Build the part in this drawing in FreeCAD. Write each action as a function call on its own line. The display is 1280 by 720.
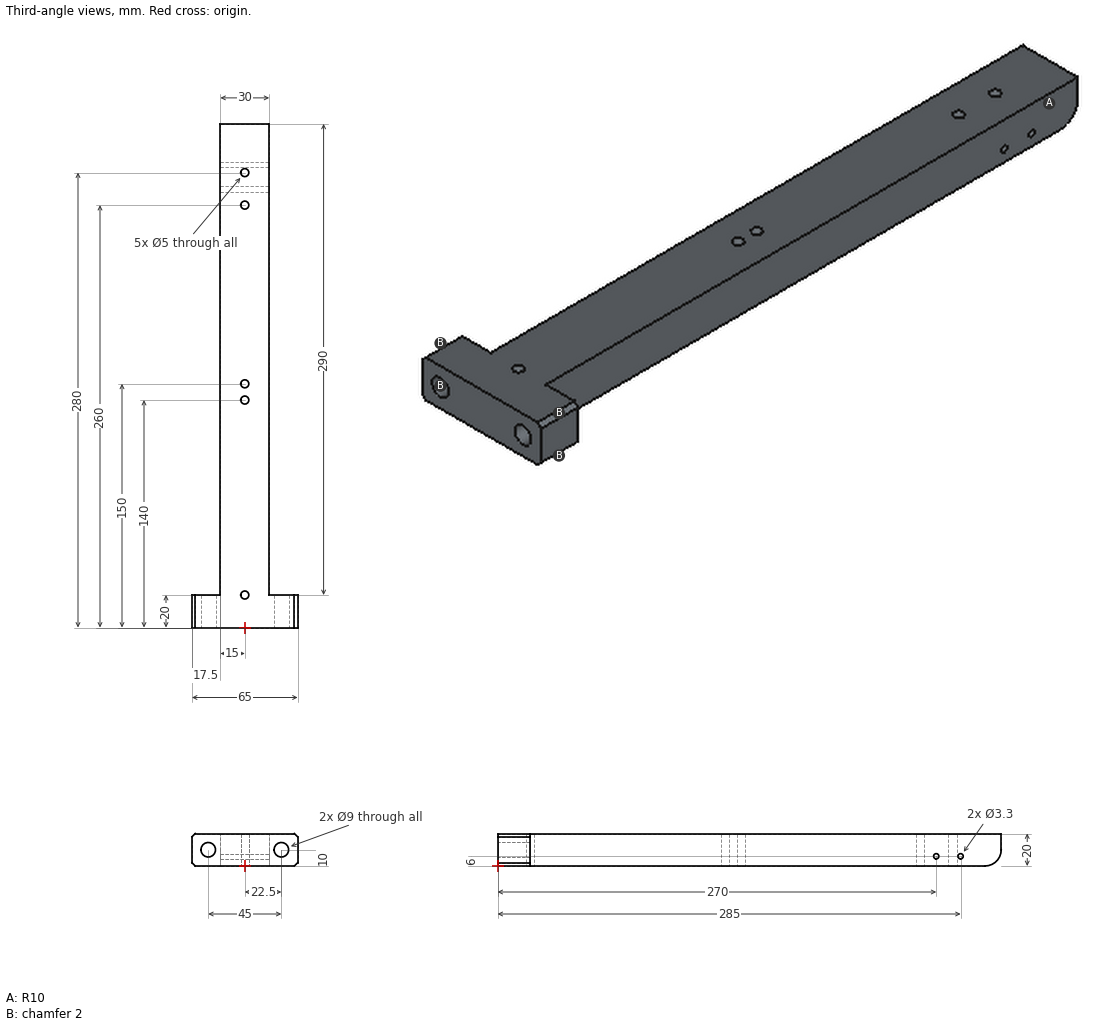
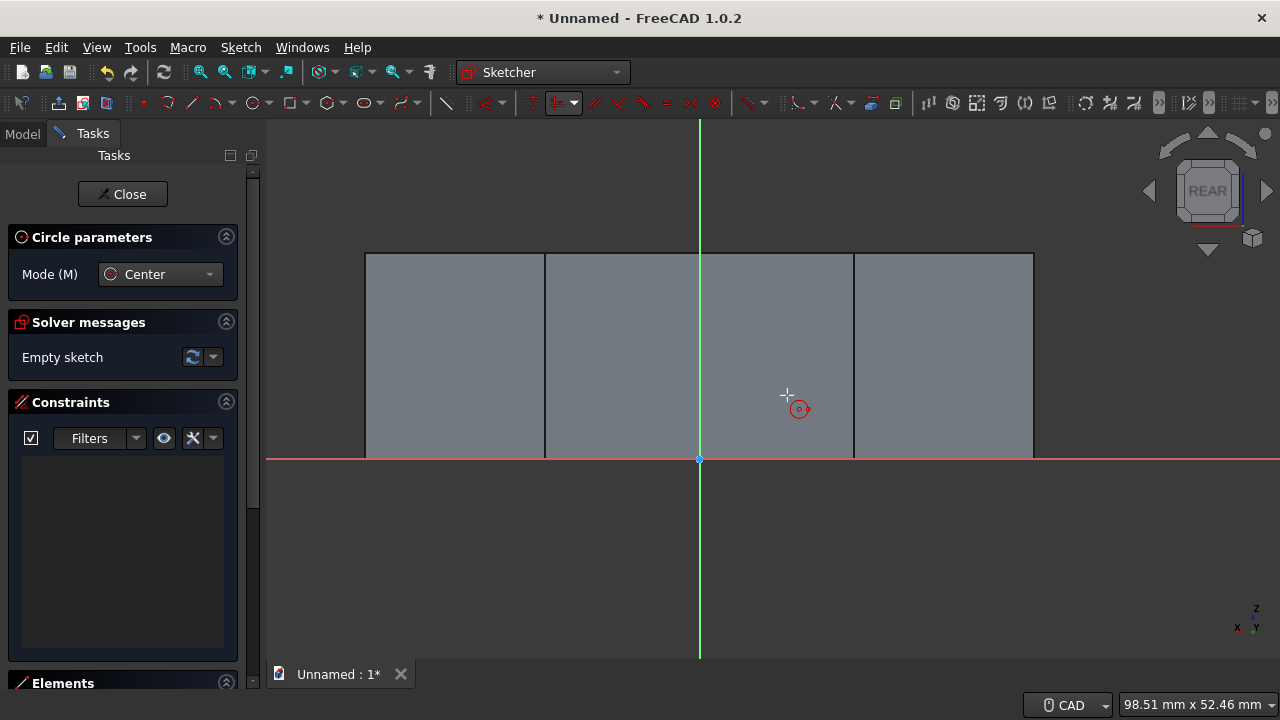
click(468, 356)
click(501, 323)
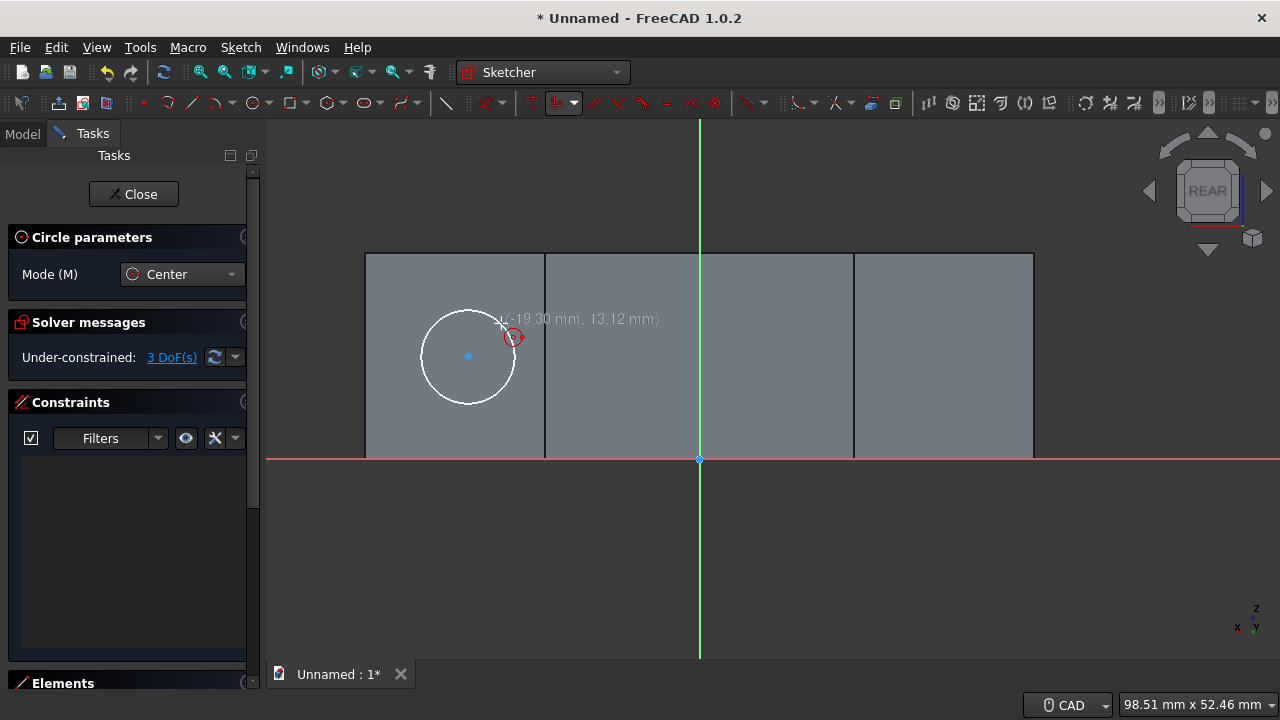
click(931, 356)
click(964, 323)
key(Escape)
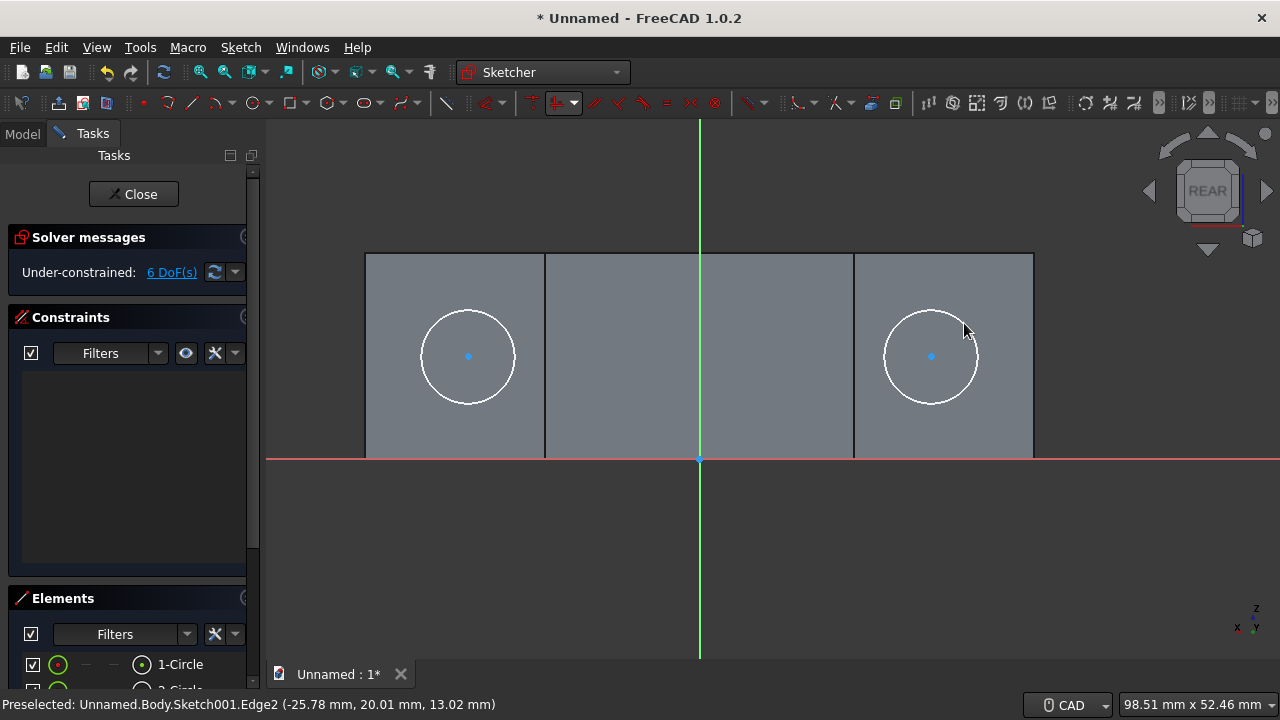
click(501, 324)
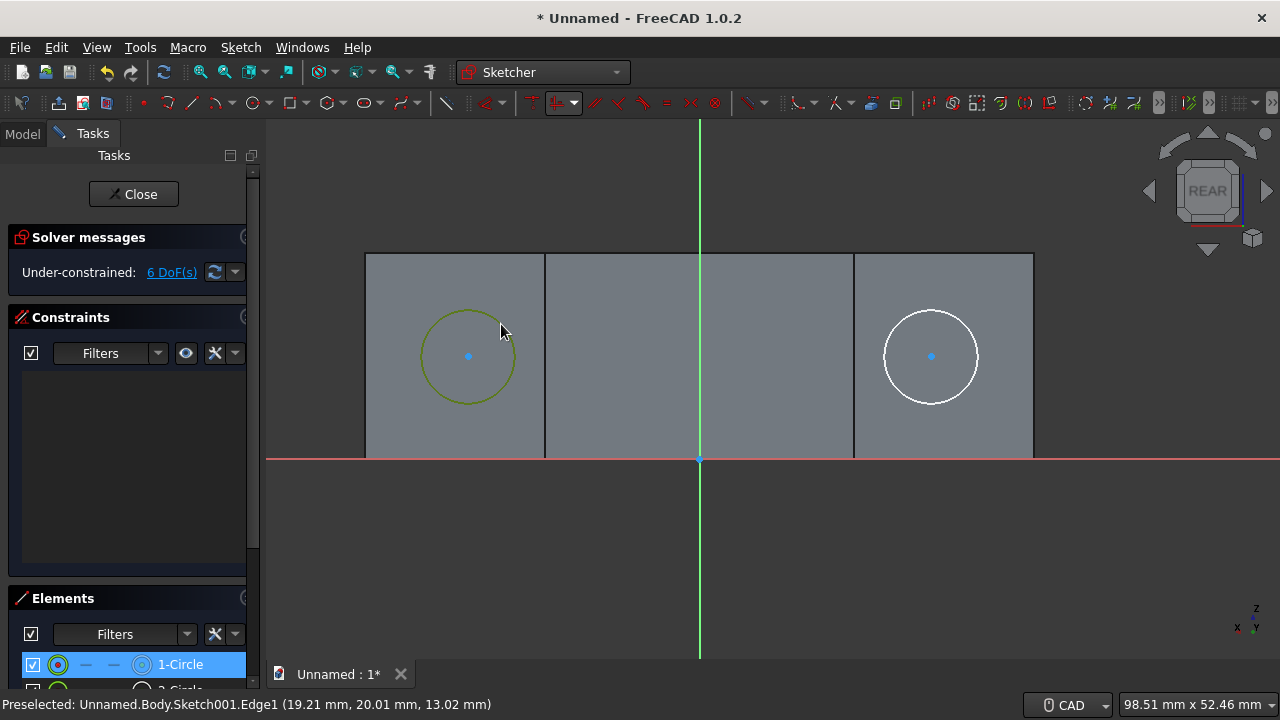
click(964, 324)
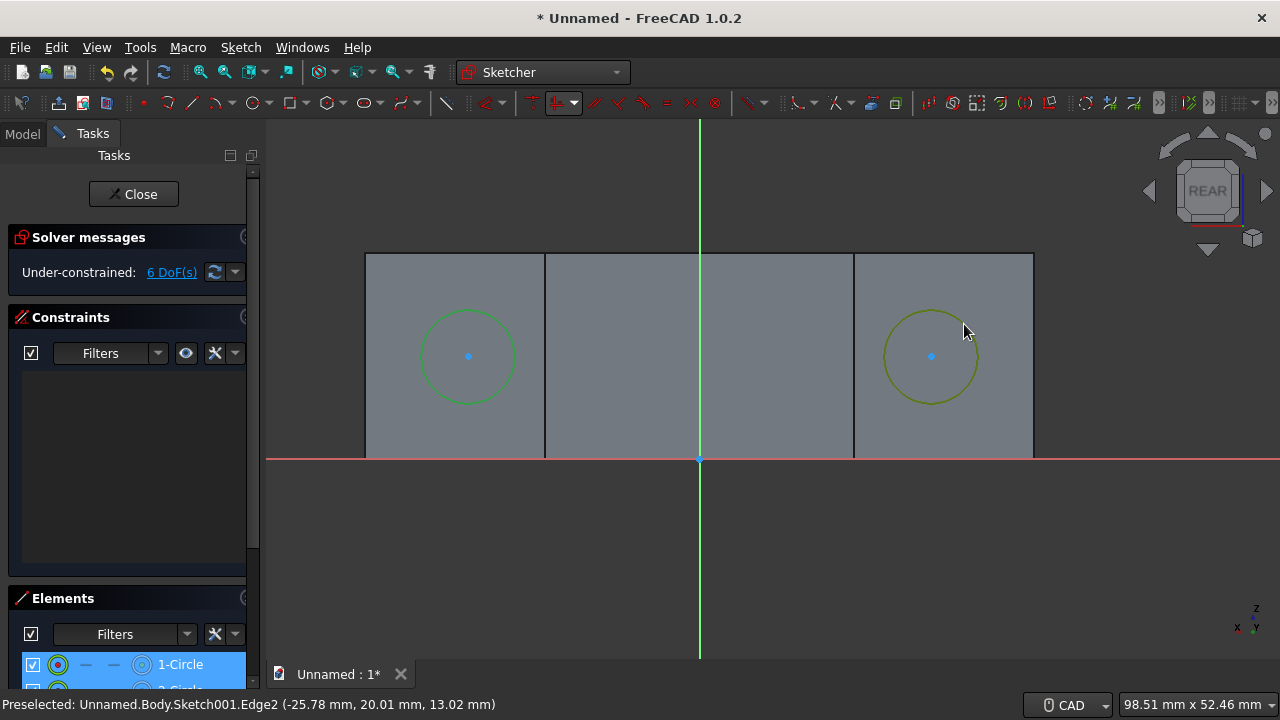
click(668, 104)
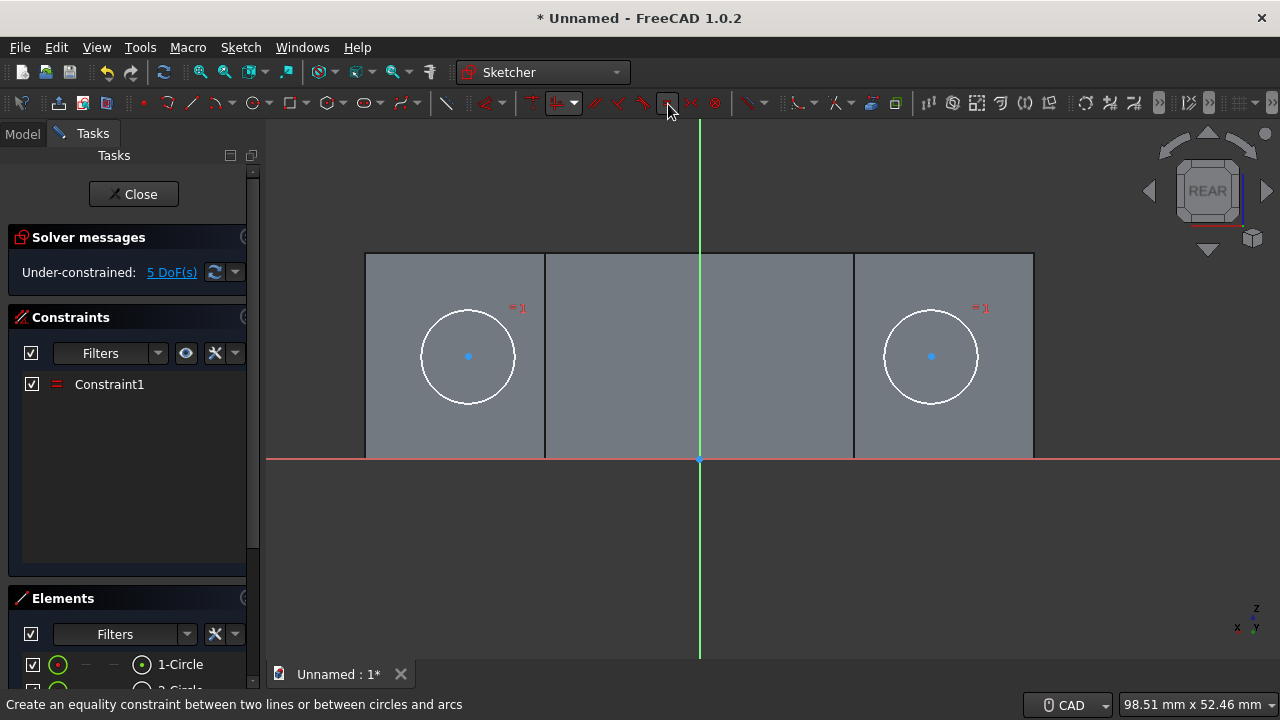
click(468, 357)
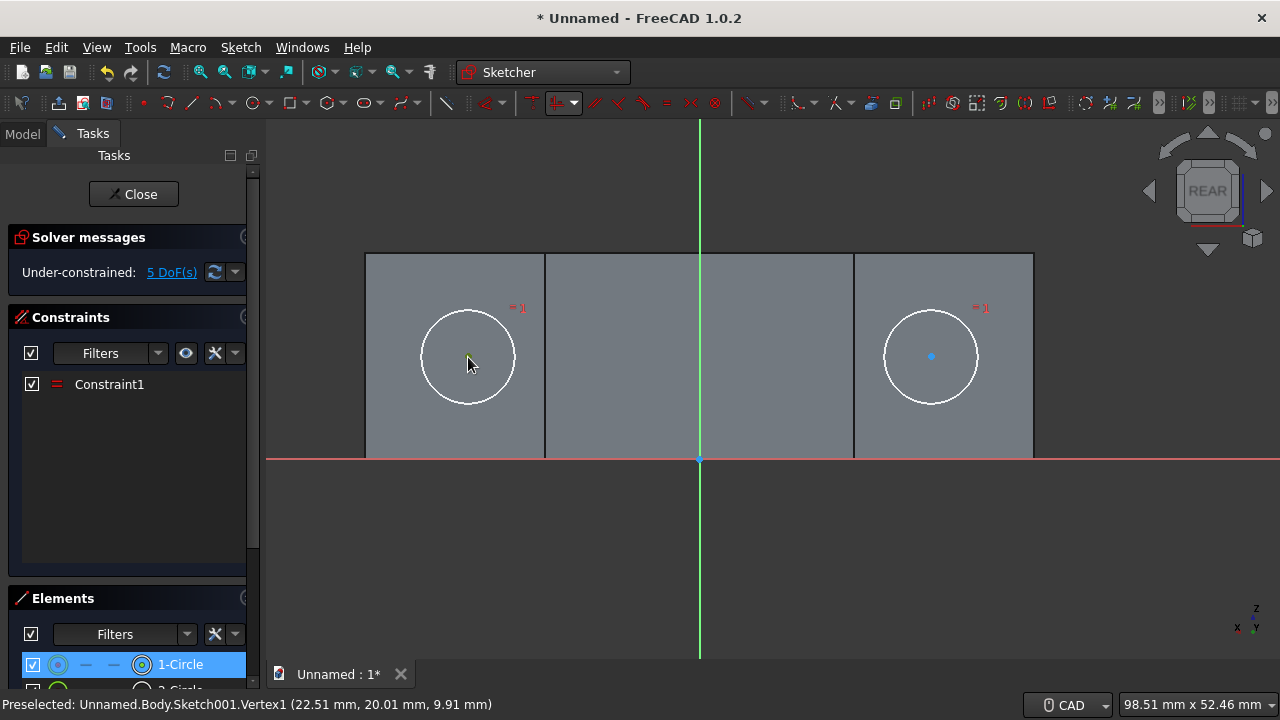
click(931, 357)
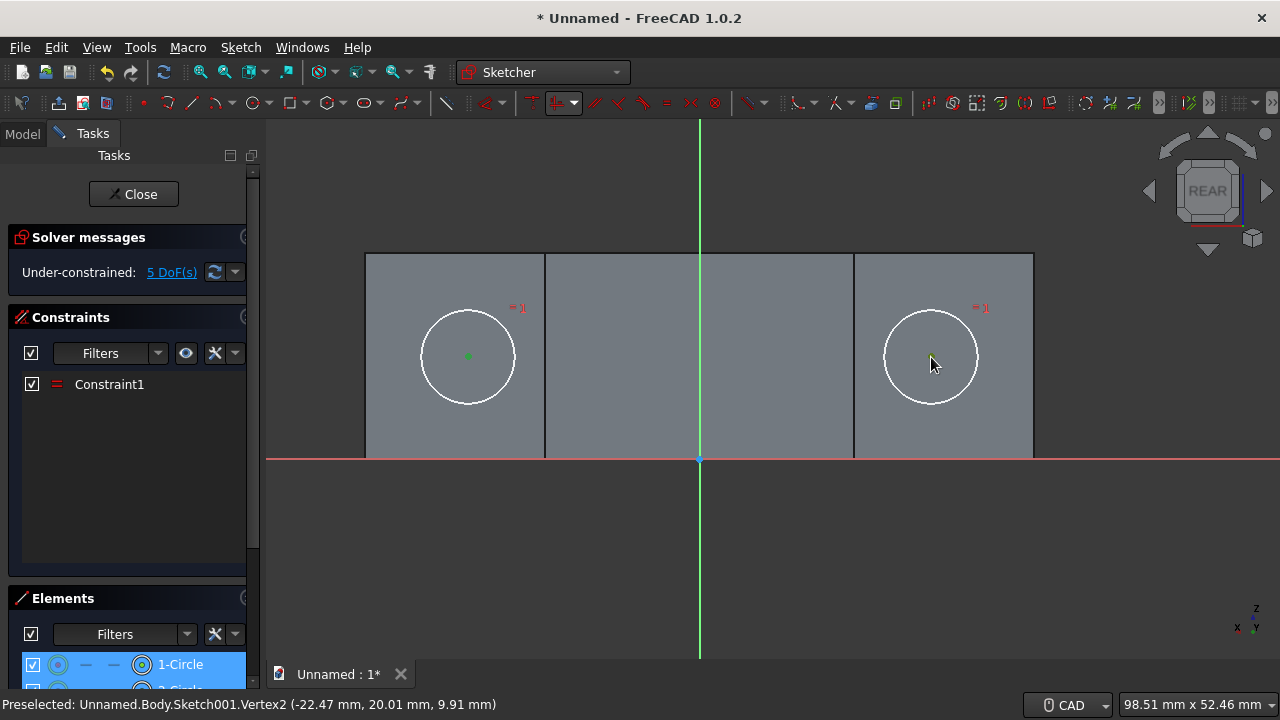
click(576, 104)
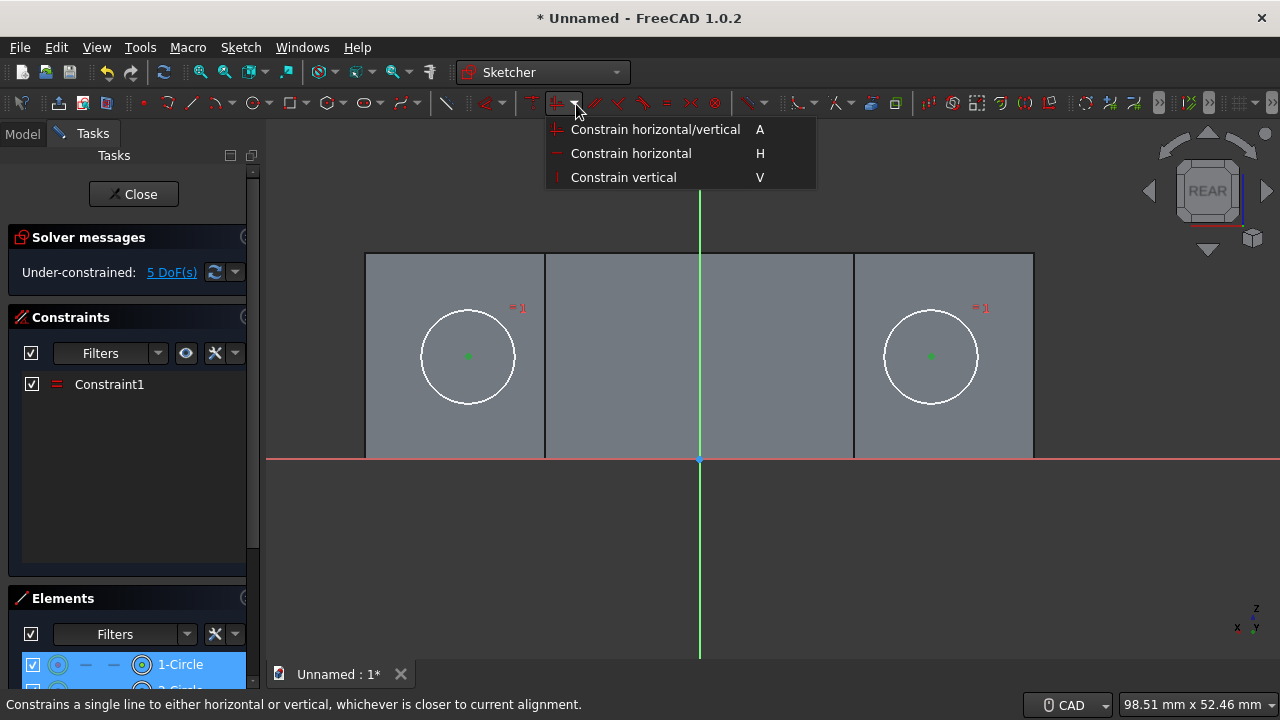
click(681, 153)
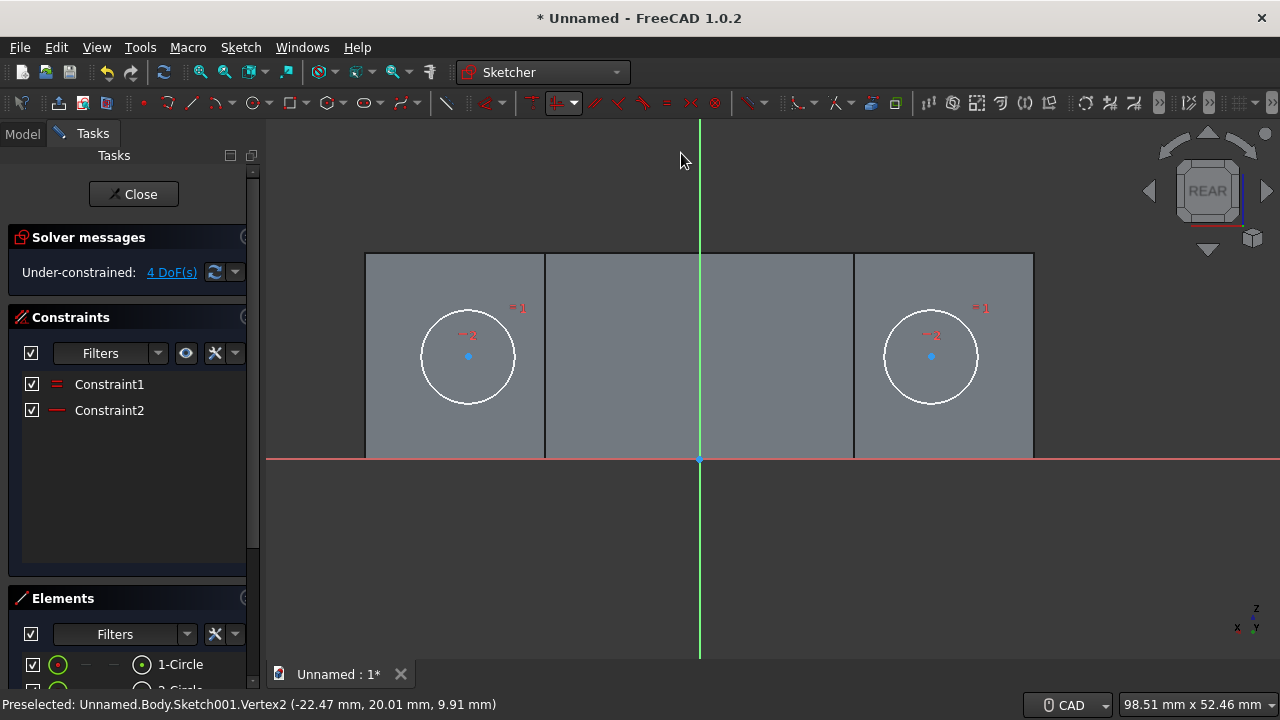
click(486, 104)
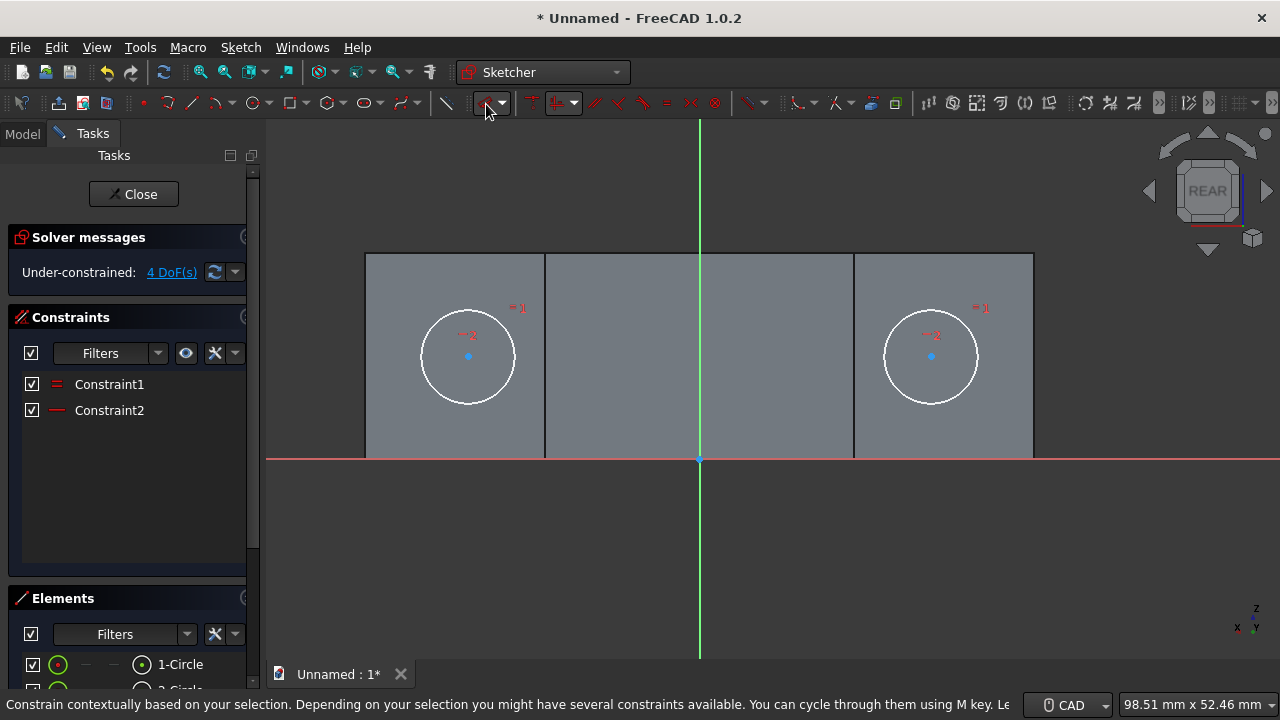
click(501, 324)
click(524, 301)